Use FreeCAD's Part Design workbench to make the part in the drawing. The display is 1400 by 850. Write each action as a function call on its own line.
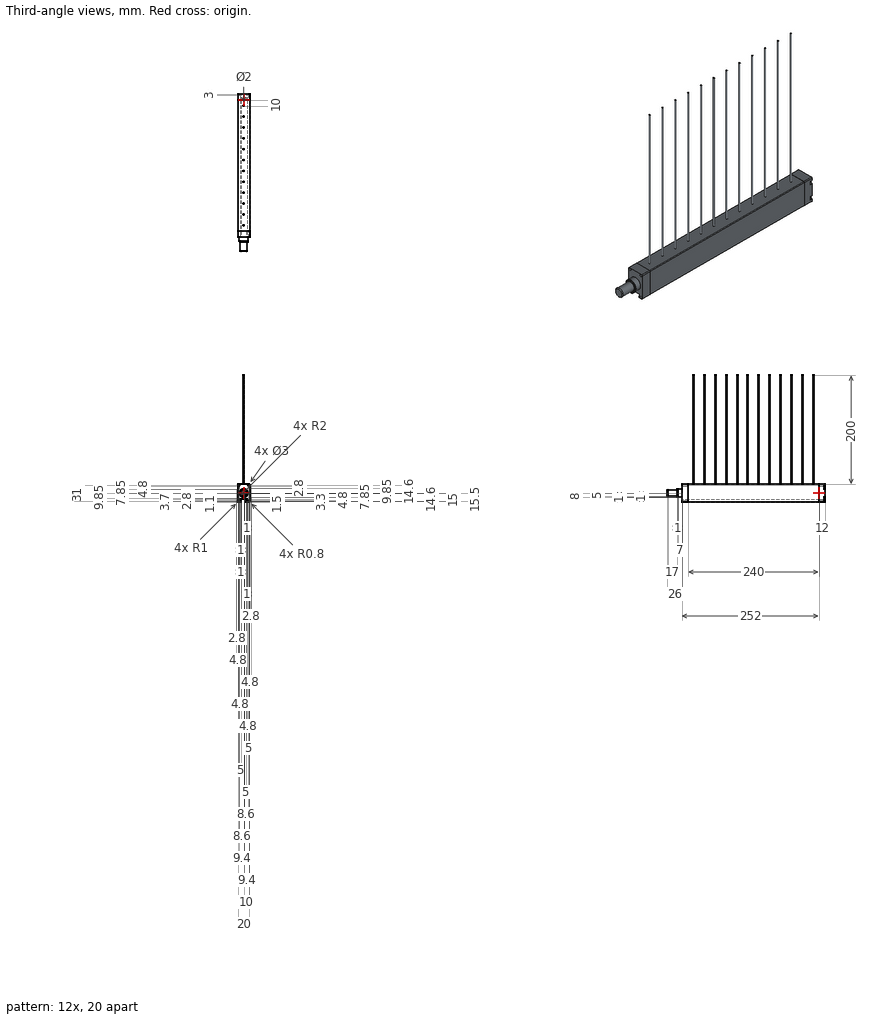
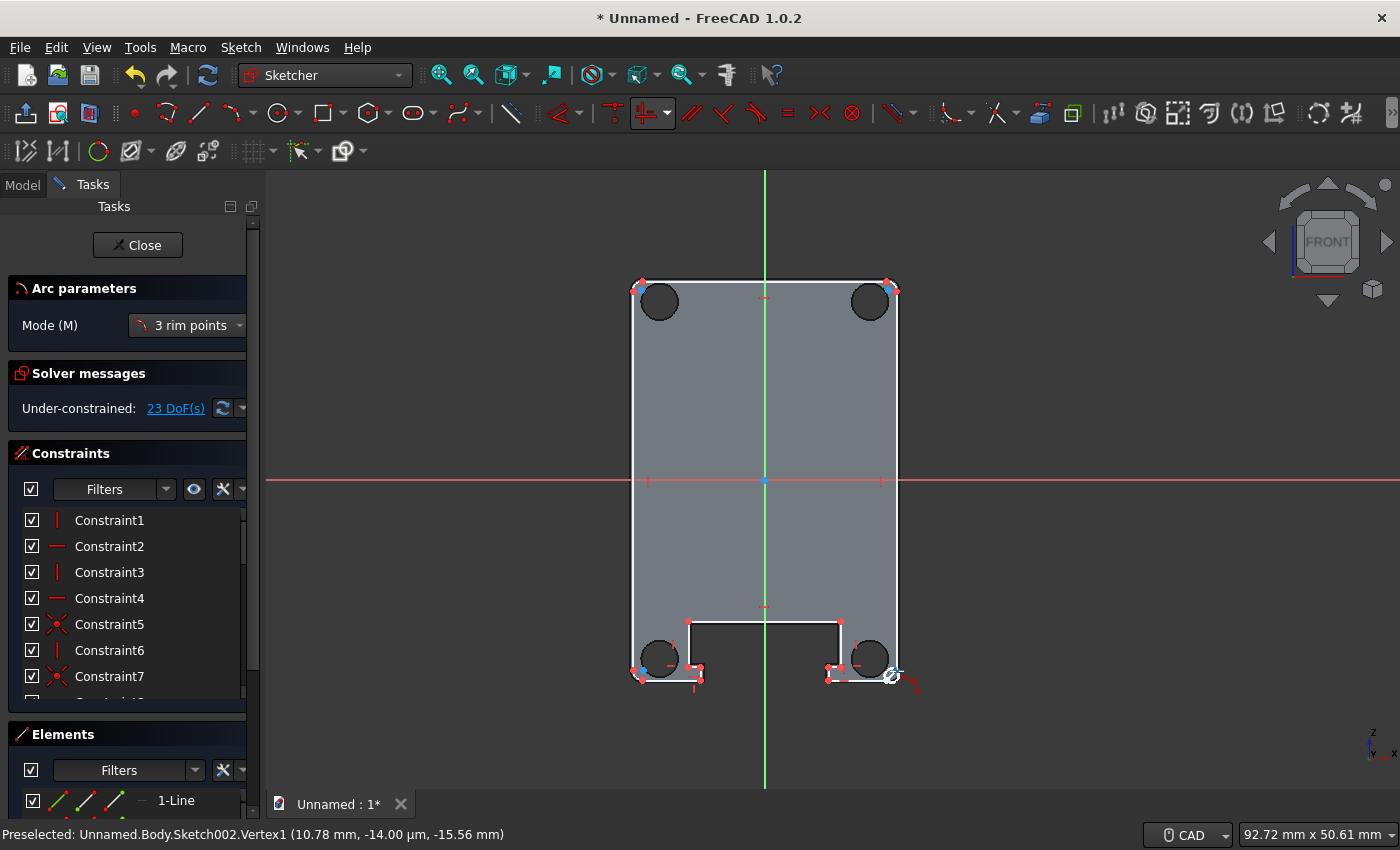
scroll(894, 677, up, 9)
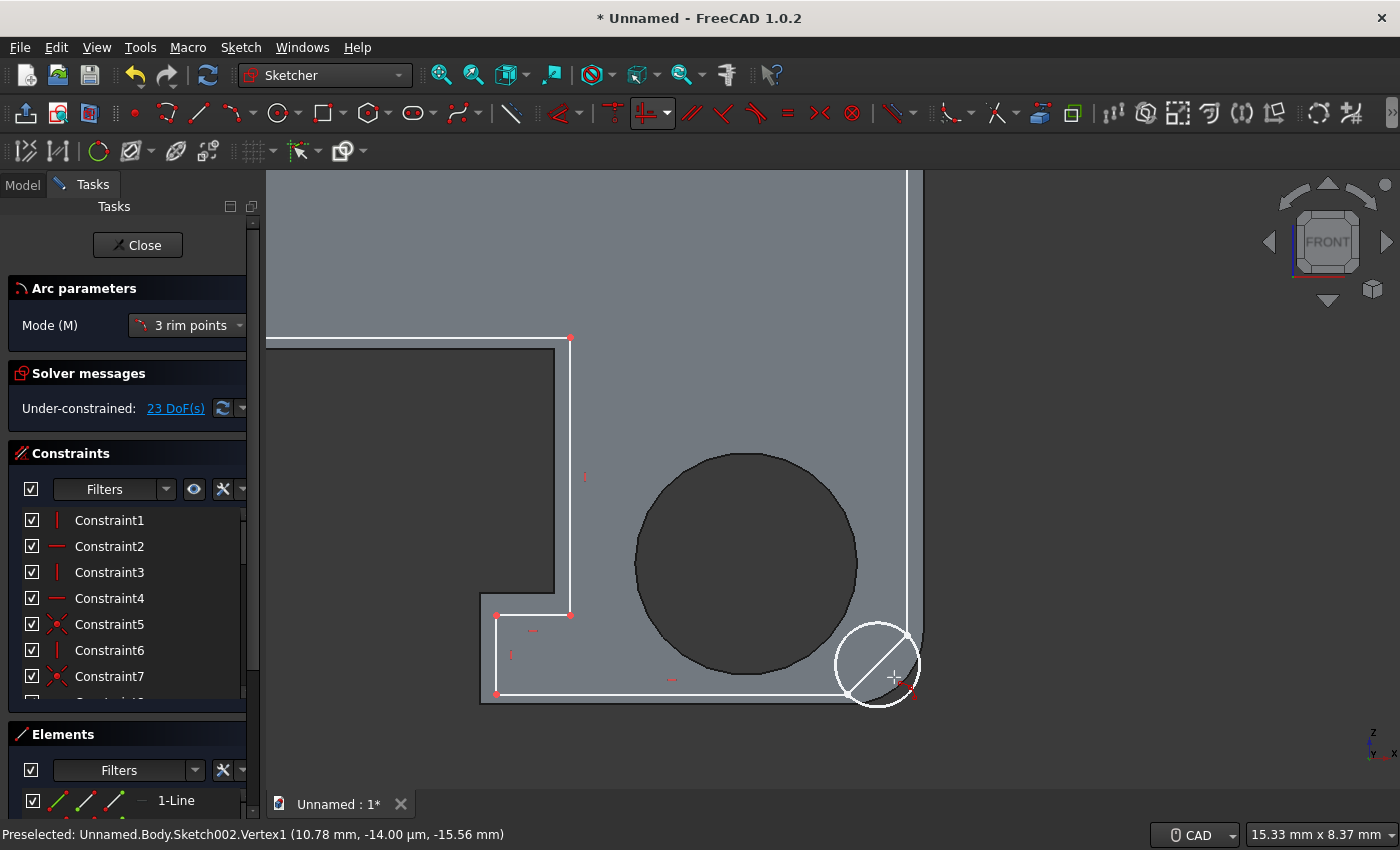
click(892, 672)
key(Escape)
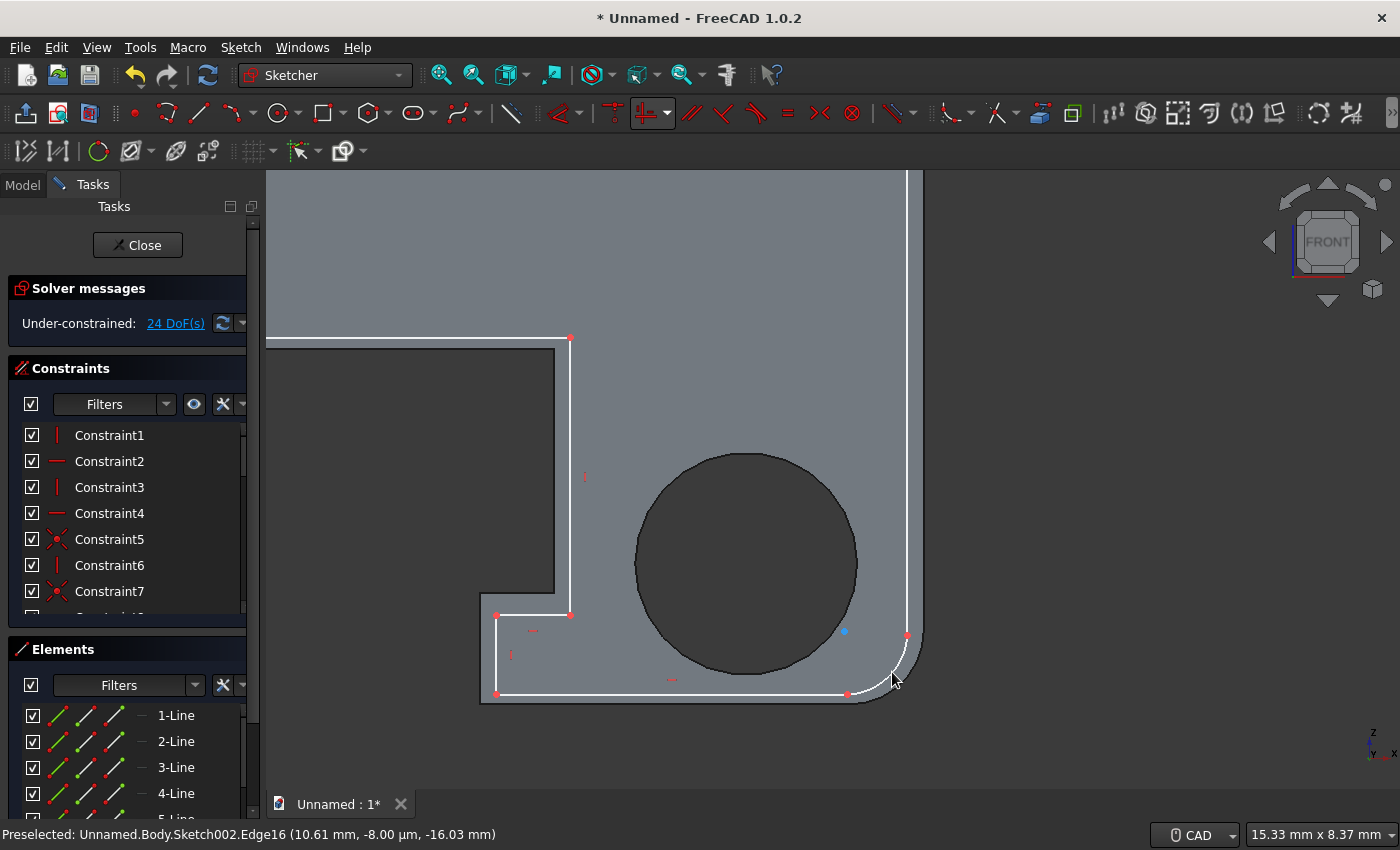
scroll(894, 677, down, 9)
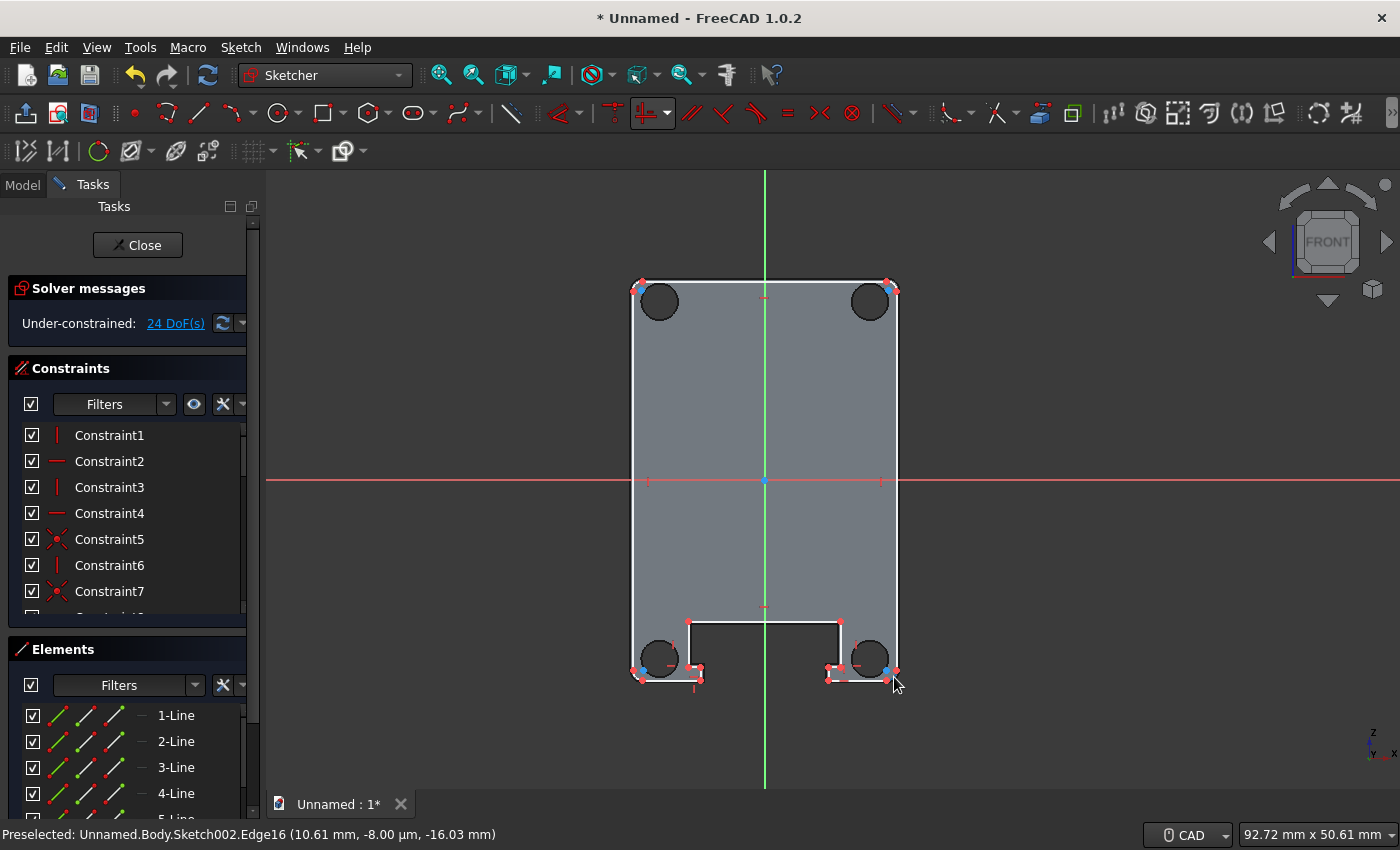
click(897, 557)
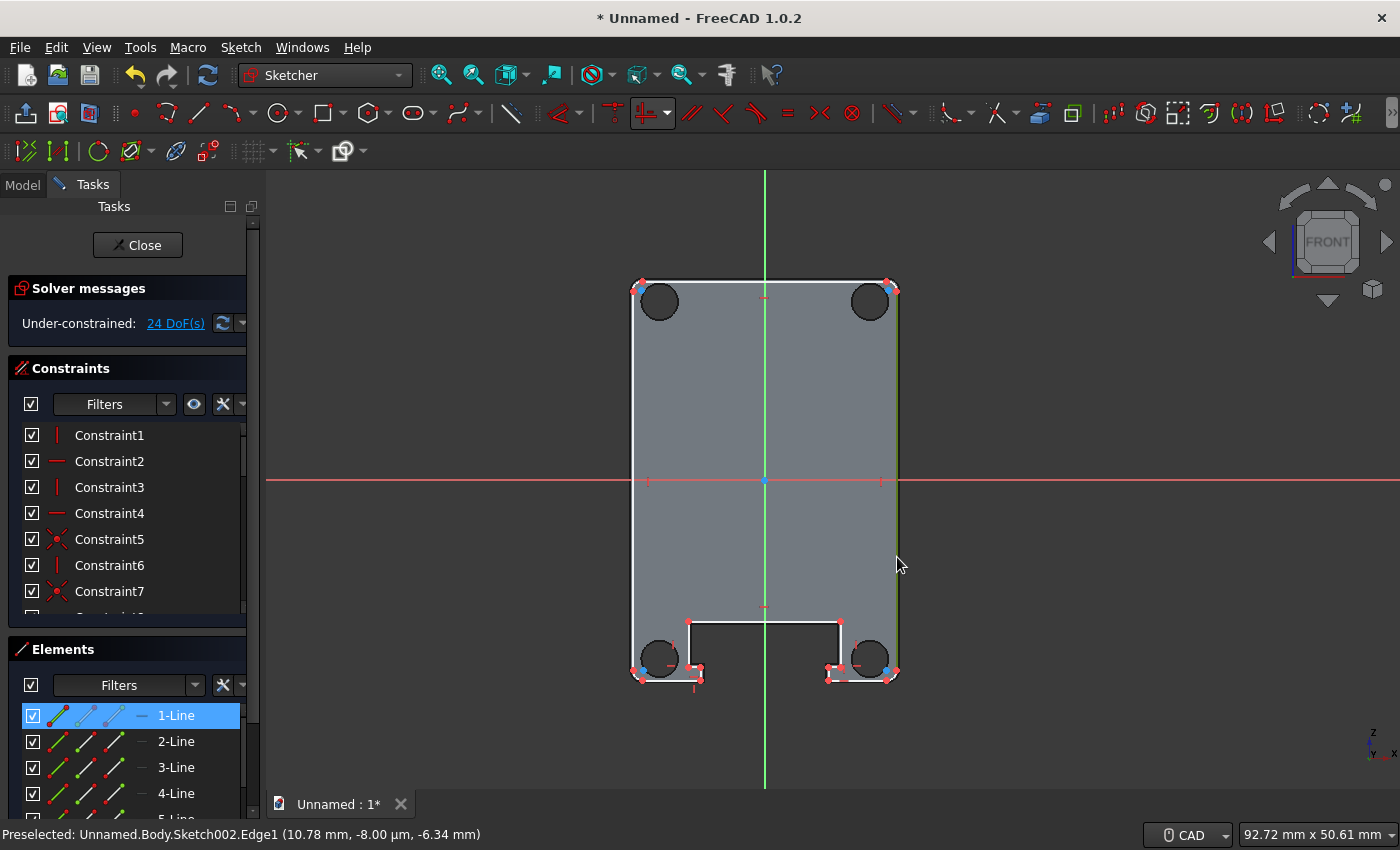
scroll(894, 284, up, 3)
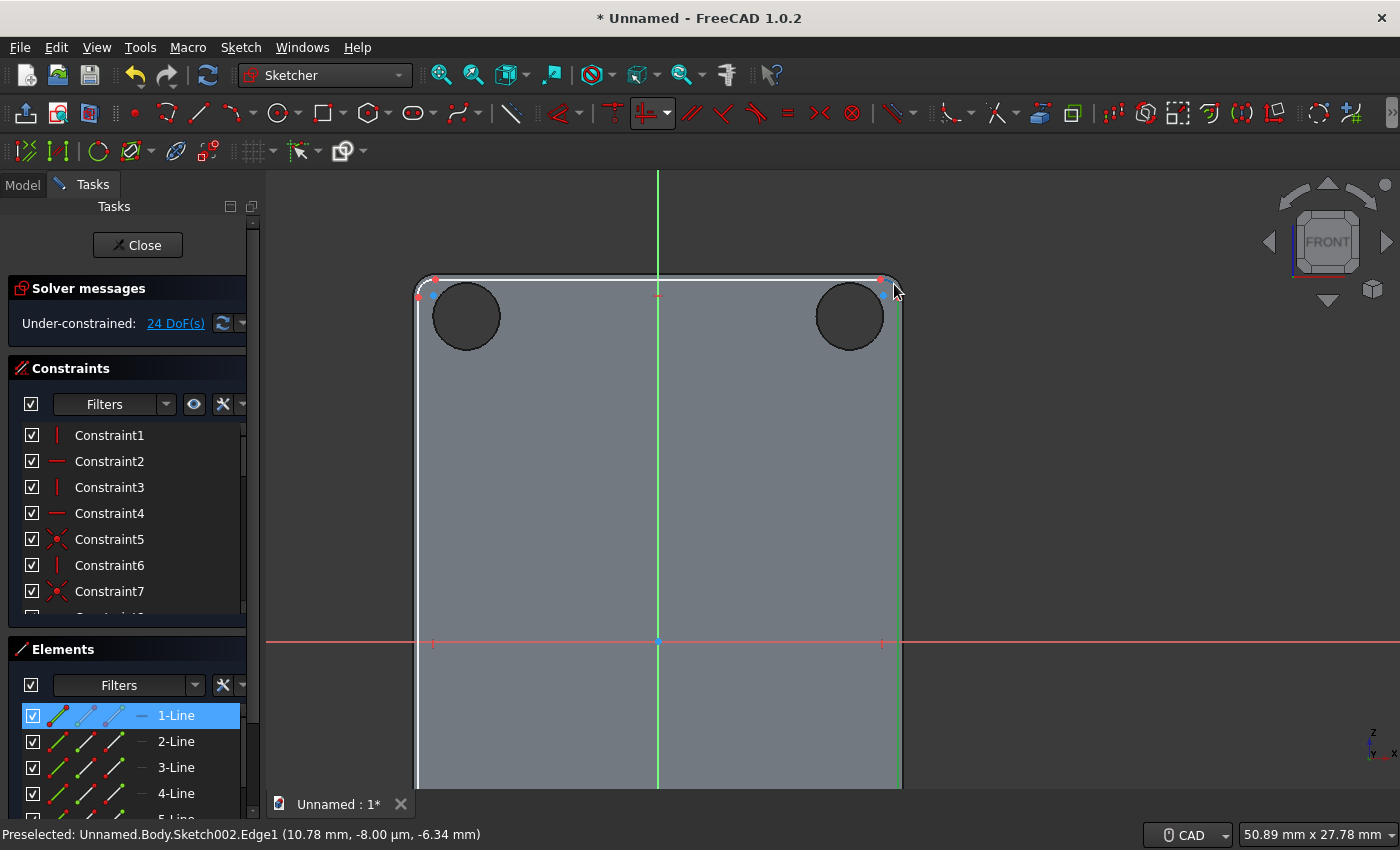
click(894, 284)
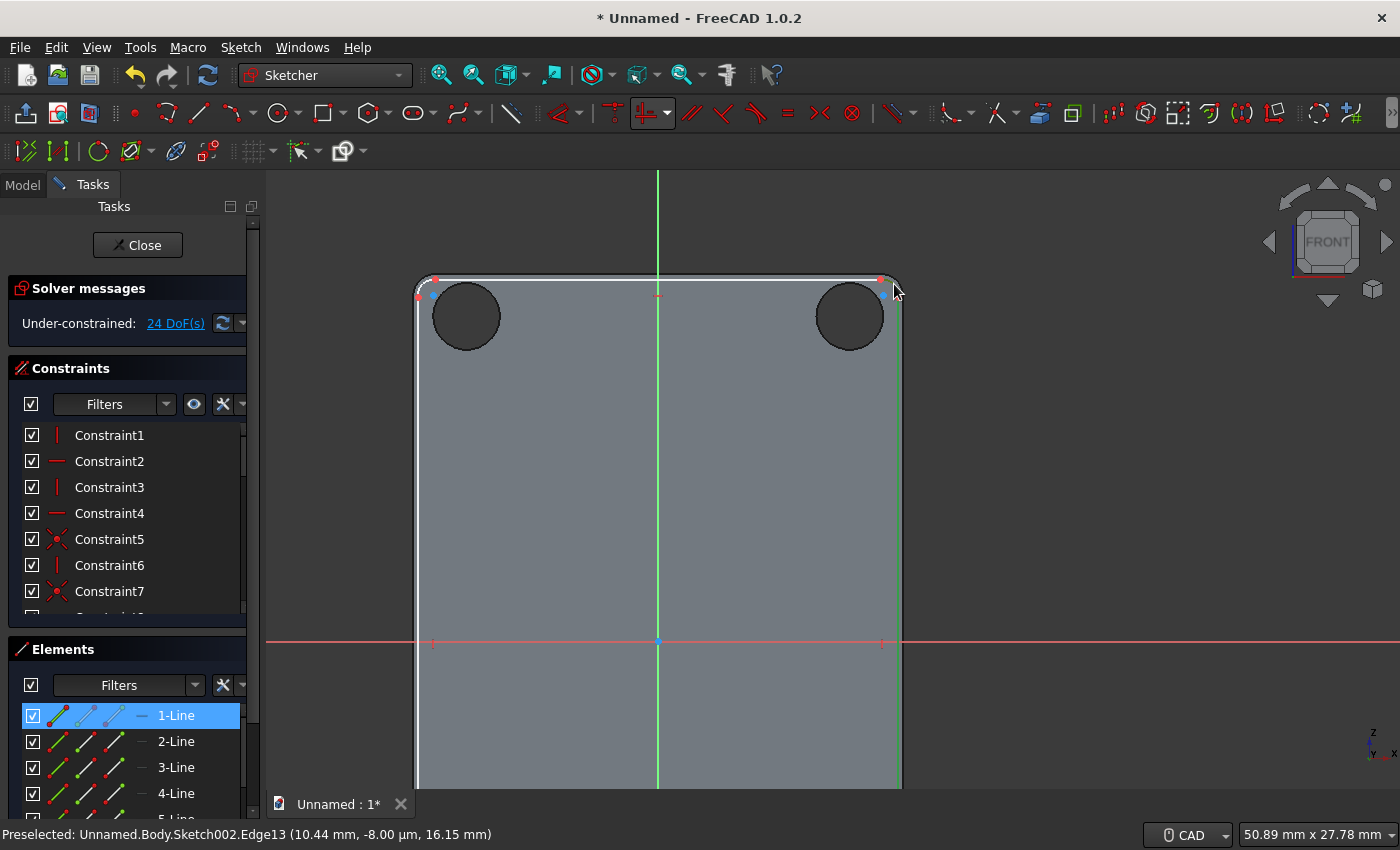
click(756, 114)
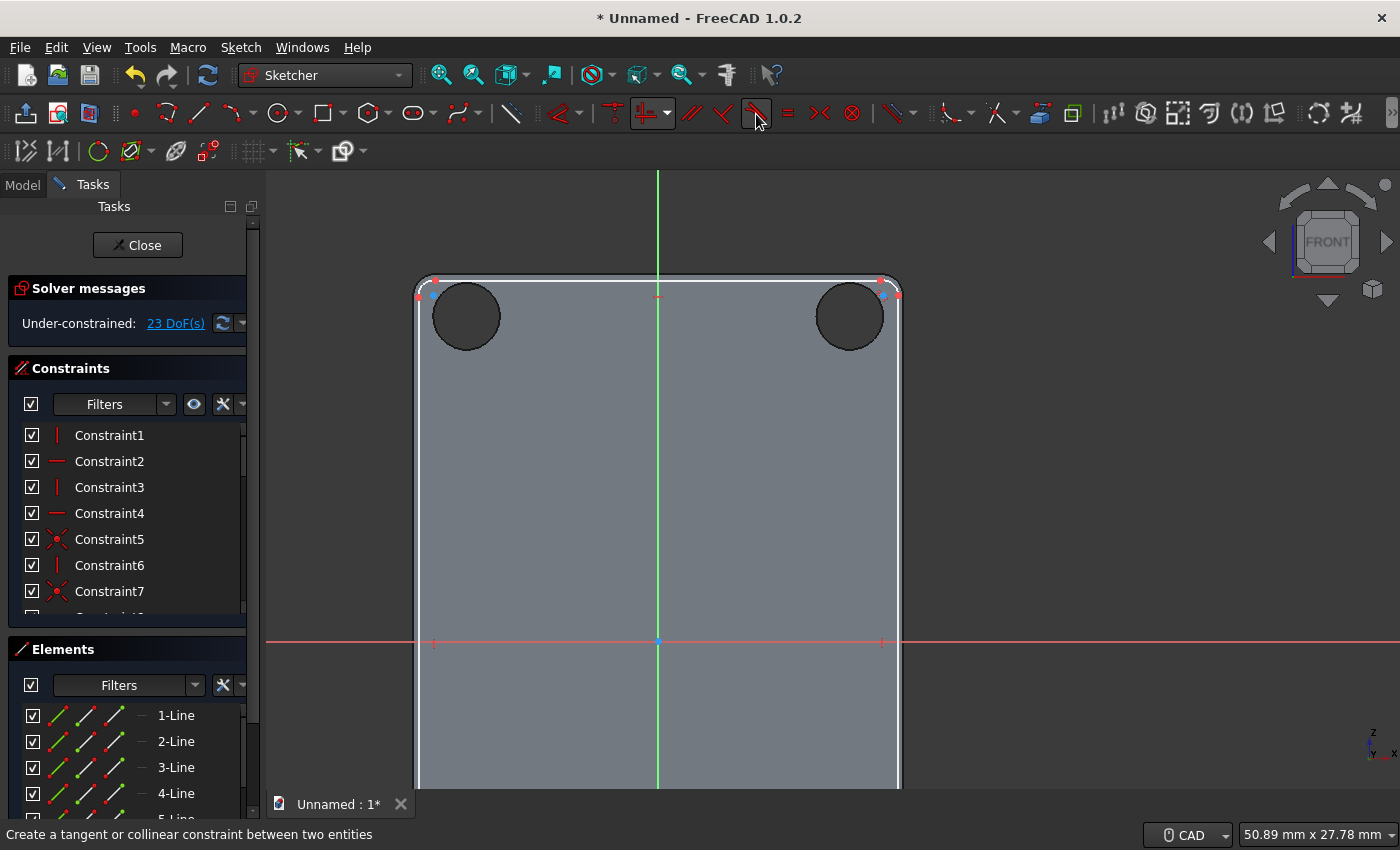
click(898, 504)